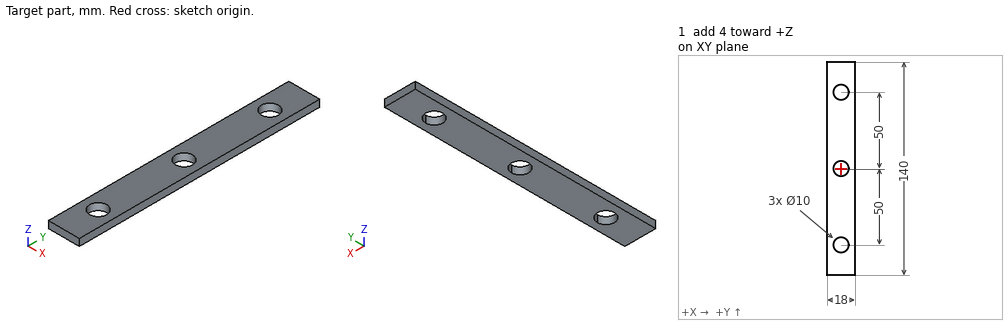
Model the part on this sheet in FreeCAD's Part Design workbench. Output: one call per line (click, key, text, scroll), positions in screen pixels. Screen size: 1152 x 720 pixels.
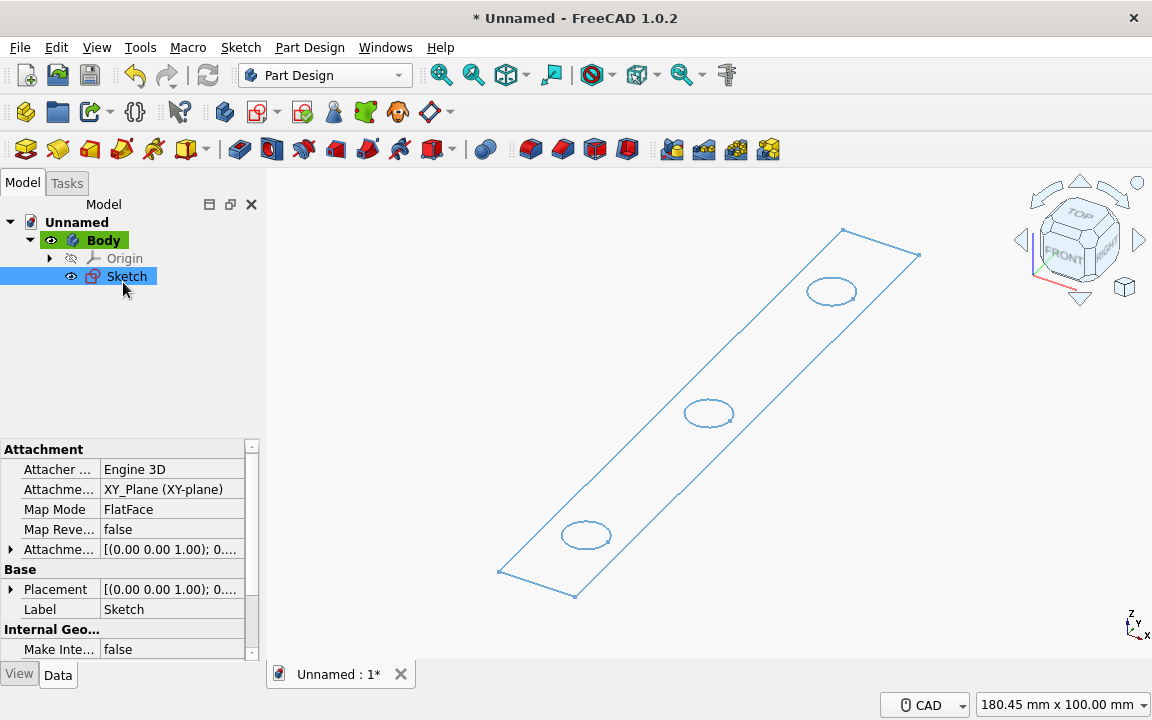
click(26, 150)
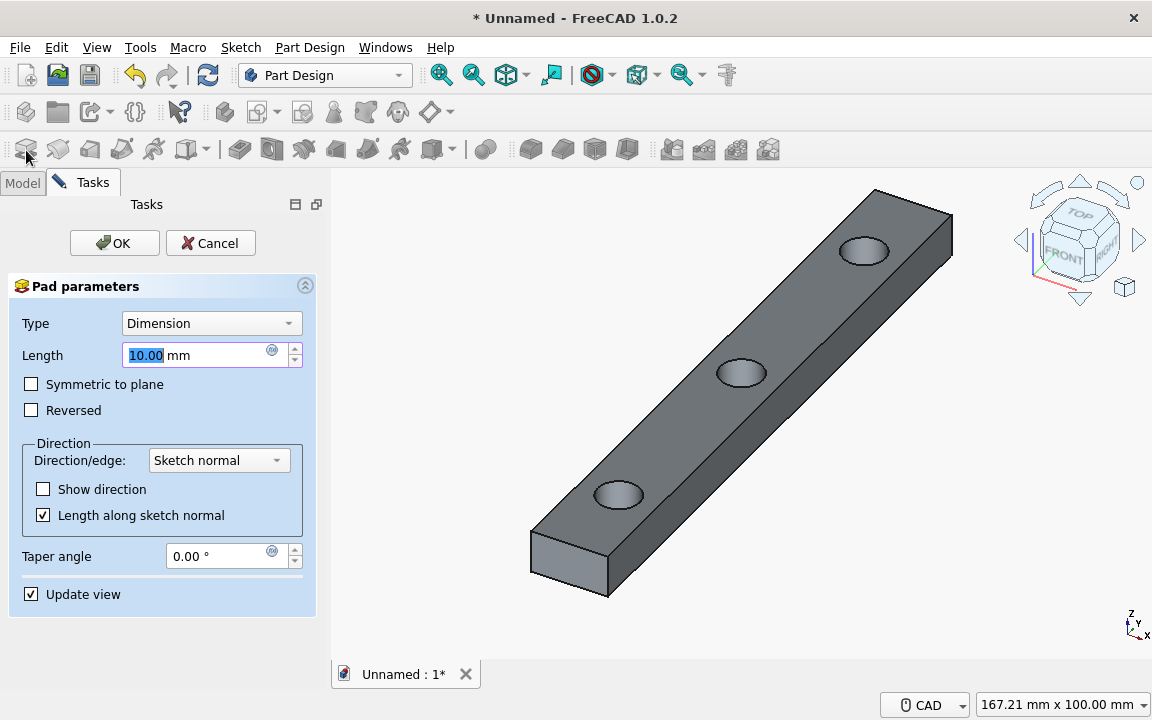
text(4)
key(Tab)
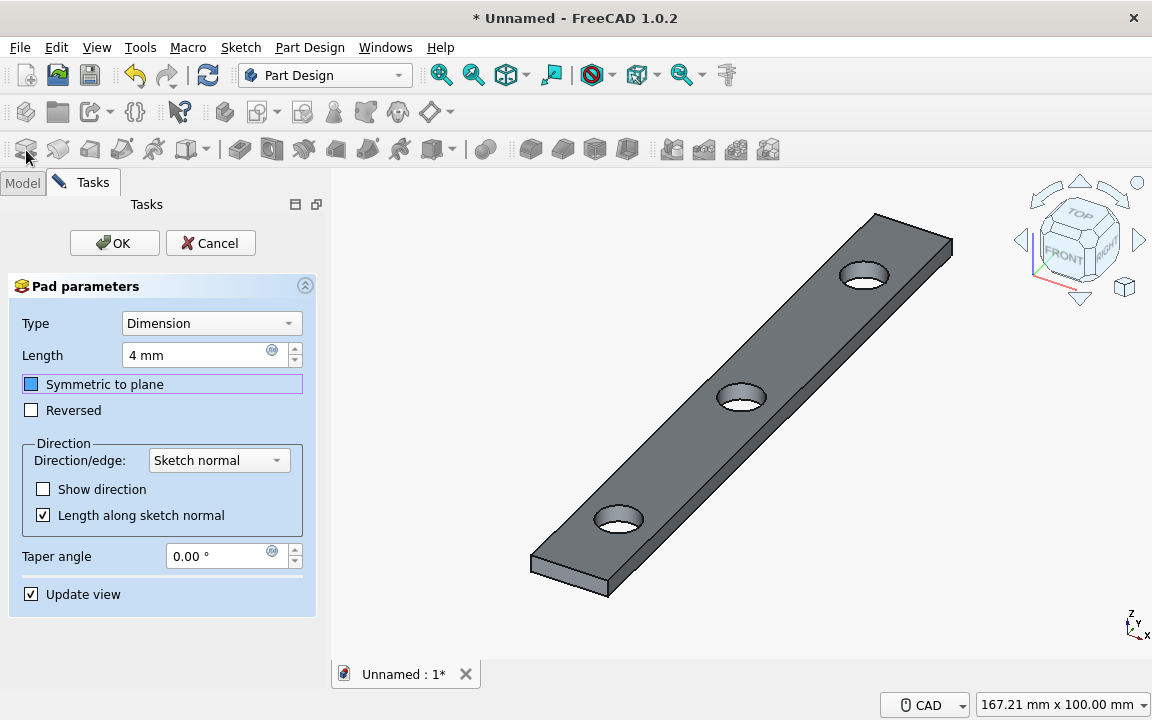
click(115, 243)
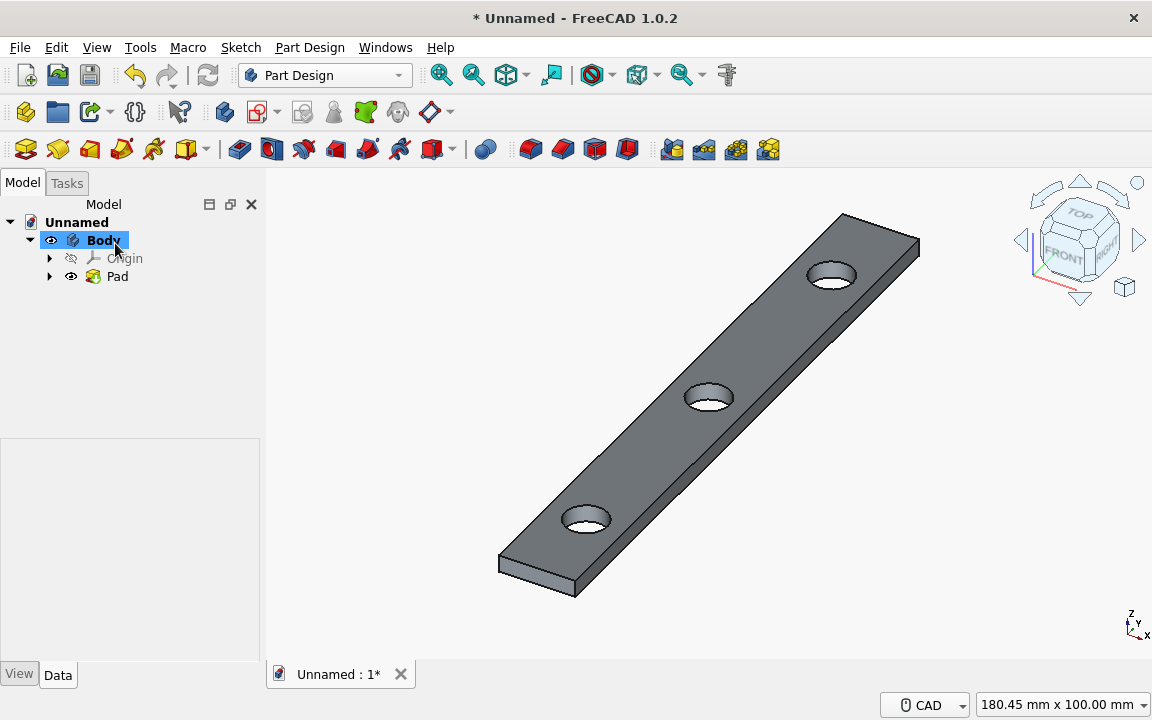
key(0)